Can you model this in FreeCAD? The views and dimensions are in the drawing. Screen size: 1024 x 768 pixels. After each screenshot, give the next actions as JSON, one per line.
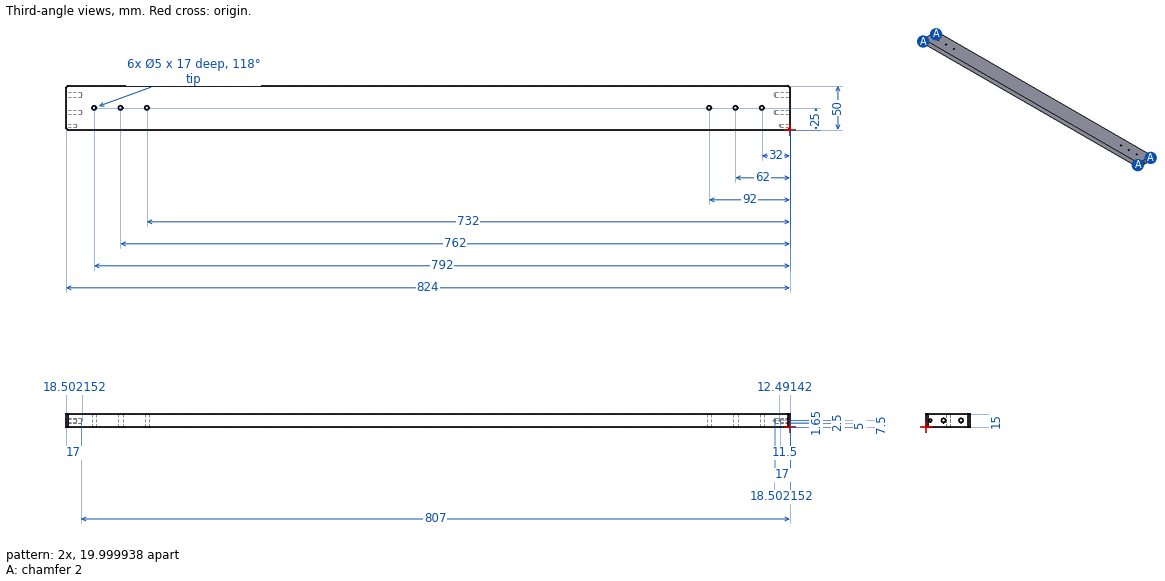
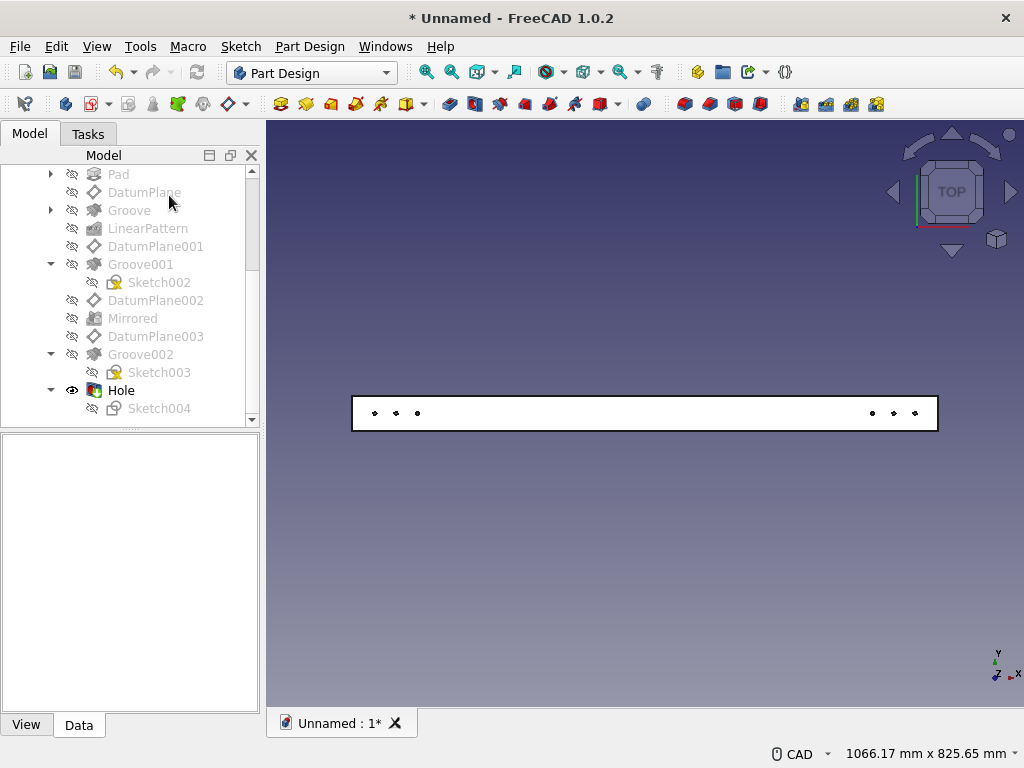
{"action": "key", "text": "1"}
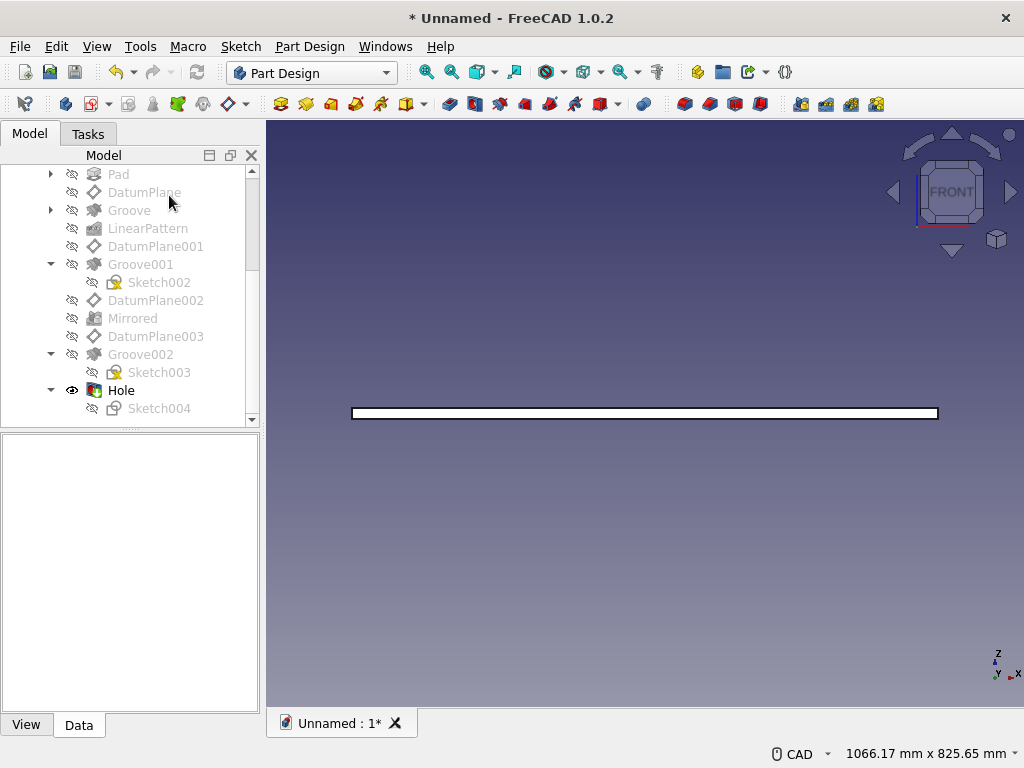
{"action": "key", "text": "3"}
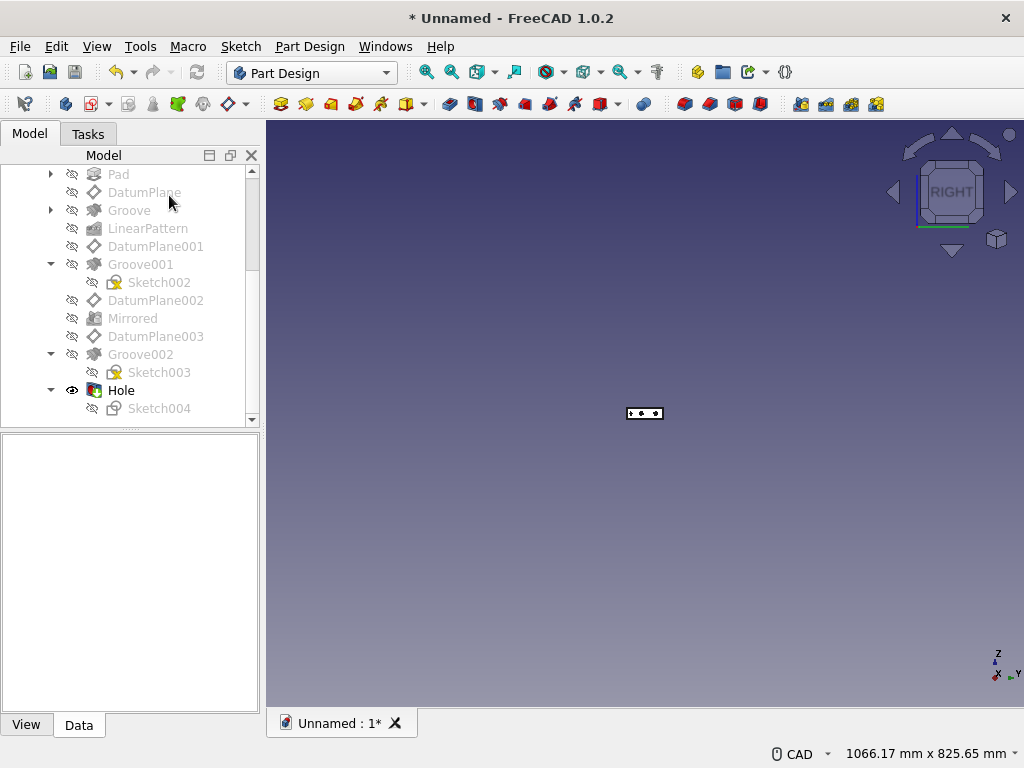
{"action": "left_click", "coordinate": [427, 72]}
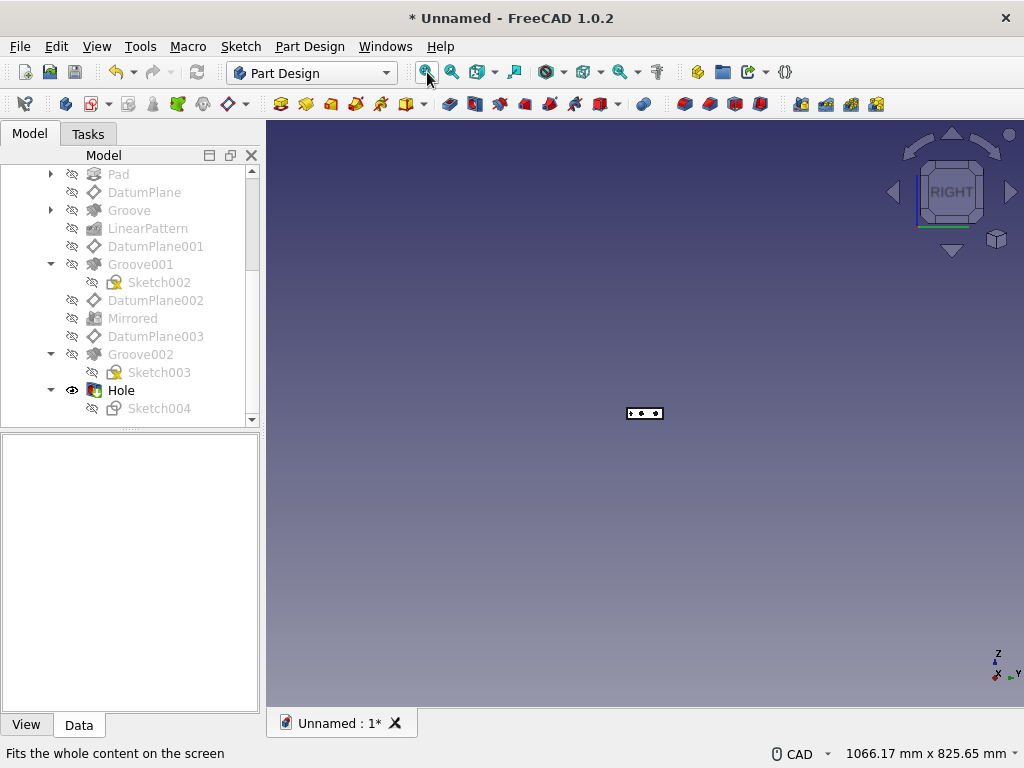
{"action": "scroll", "coordinate": [663, 412], "scroll_direction": "up", "scroll_amount": 7}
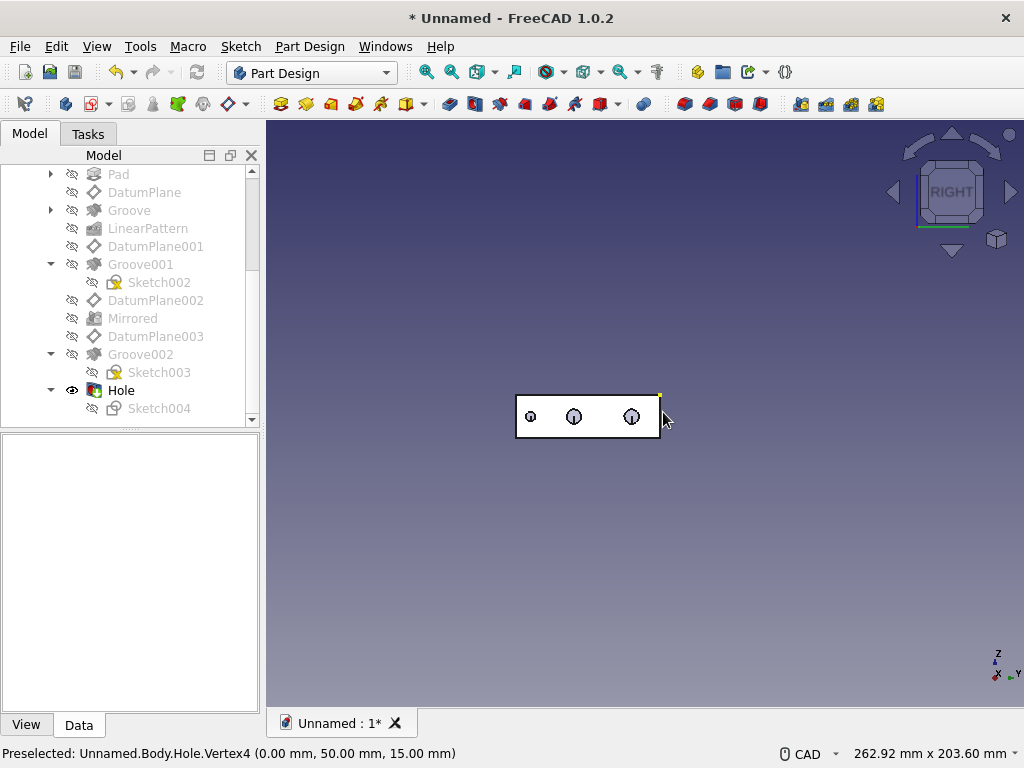
{"action": "left_click", "coordinate": [660, 416]}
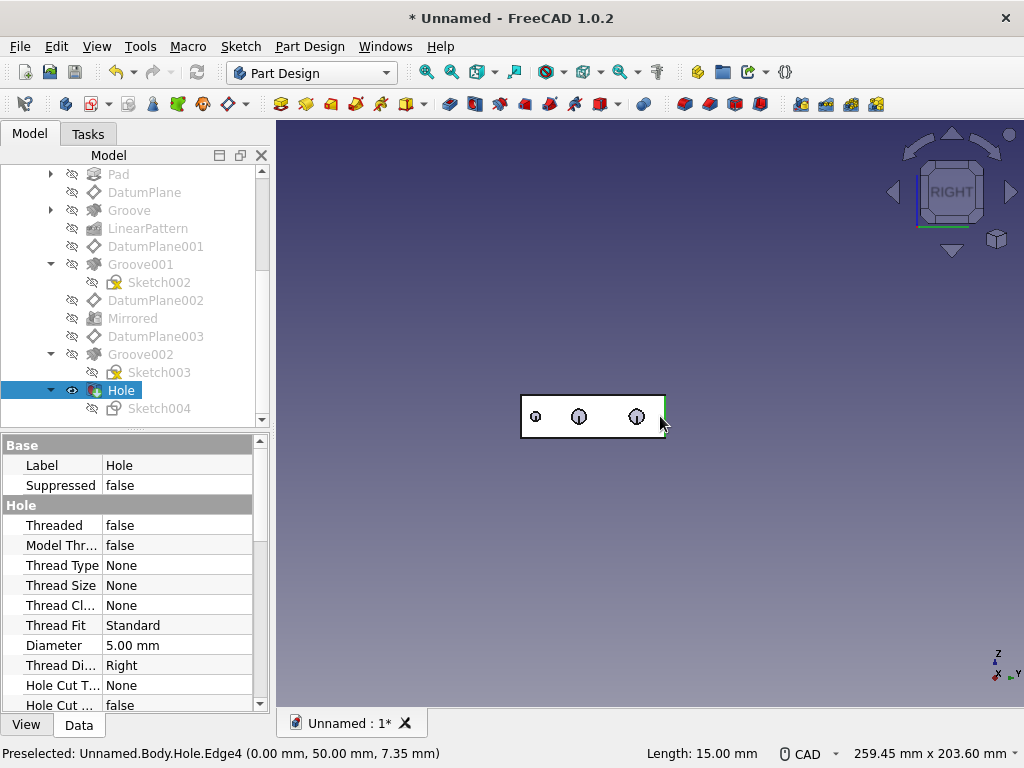
{"action": "left_click", "coordinate": [521, 416], "text": "ctrl"}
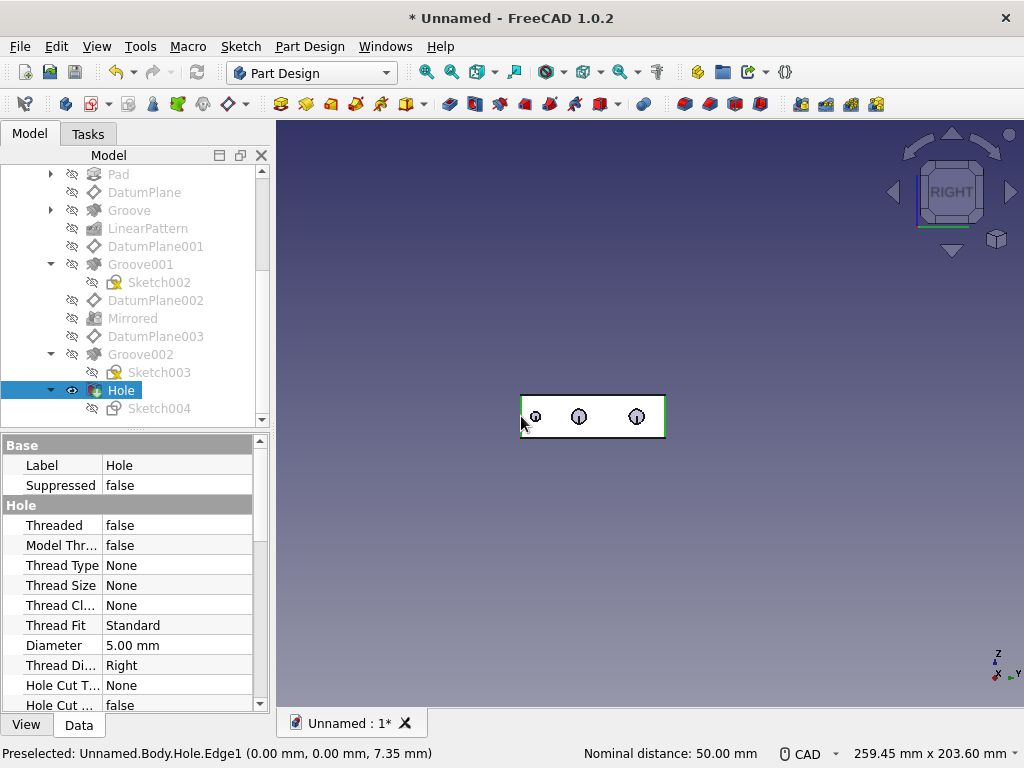
{"action": "left_click", "coordinate": [427, 72]}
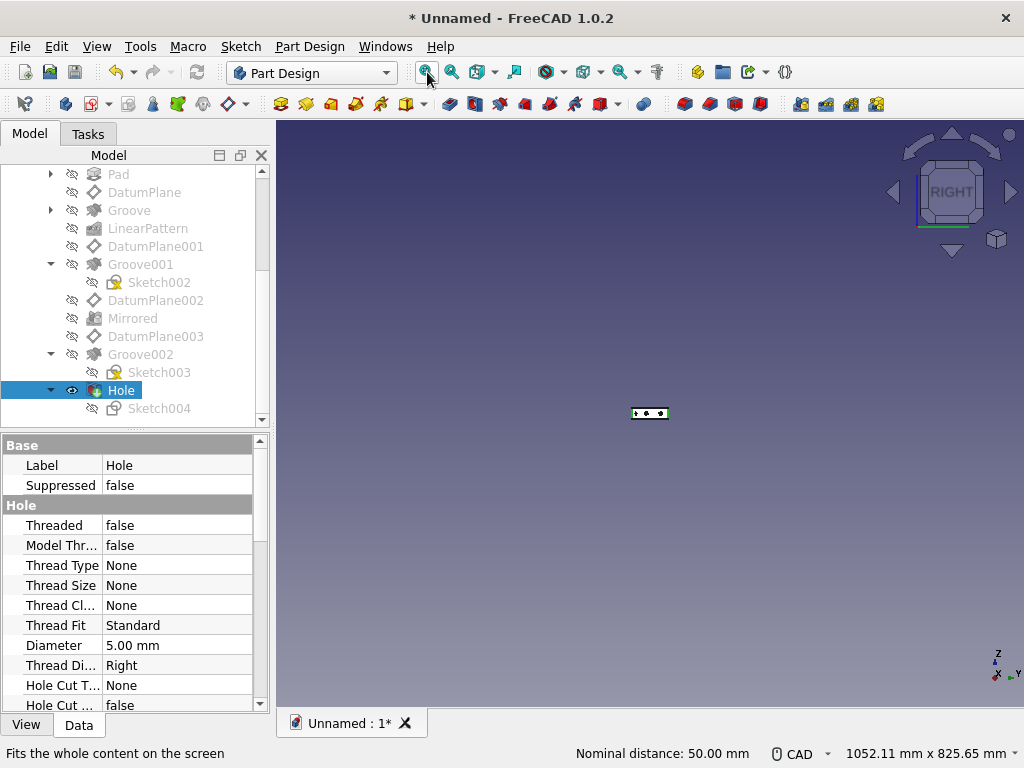
{"action": "key", "text": "5"}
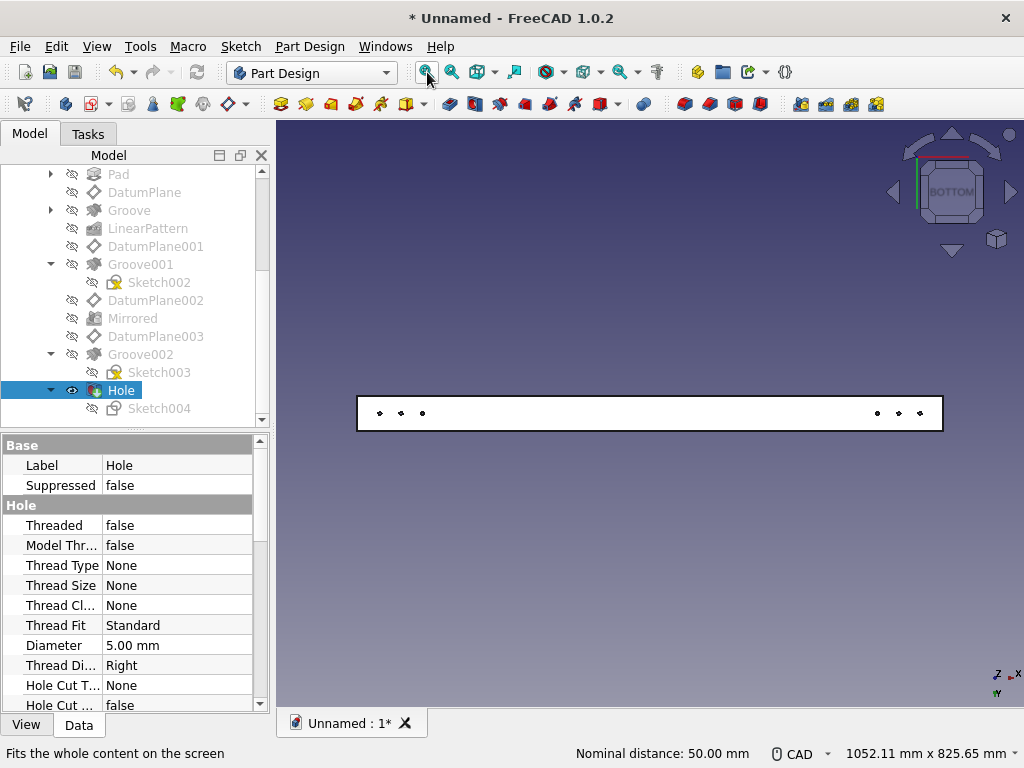
{"action": "scroll", "coordinate": [357, 395], "scroll_direction": "up", "scroll_amount": 7}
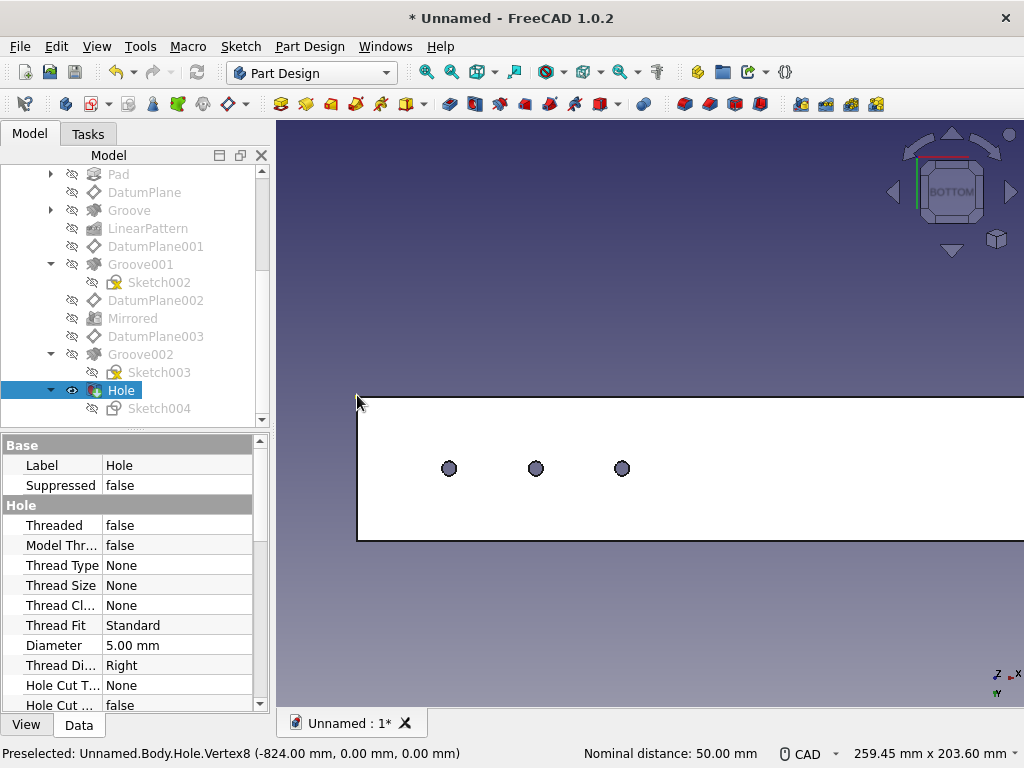
{"action": "left_click", "coordinate": [427, 72]}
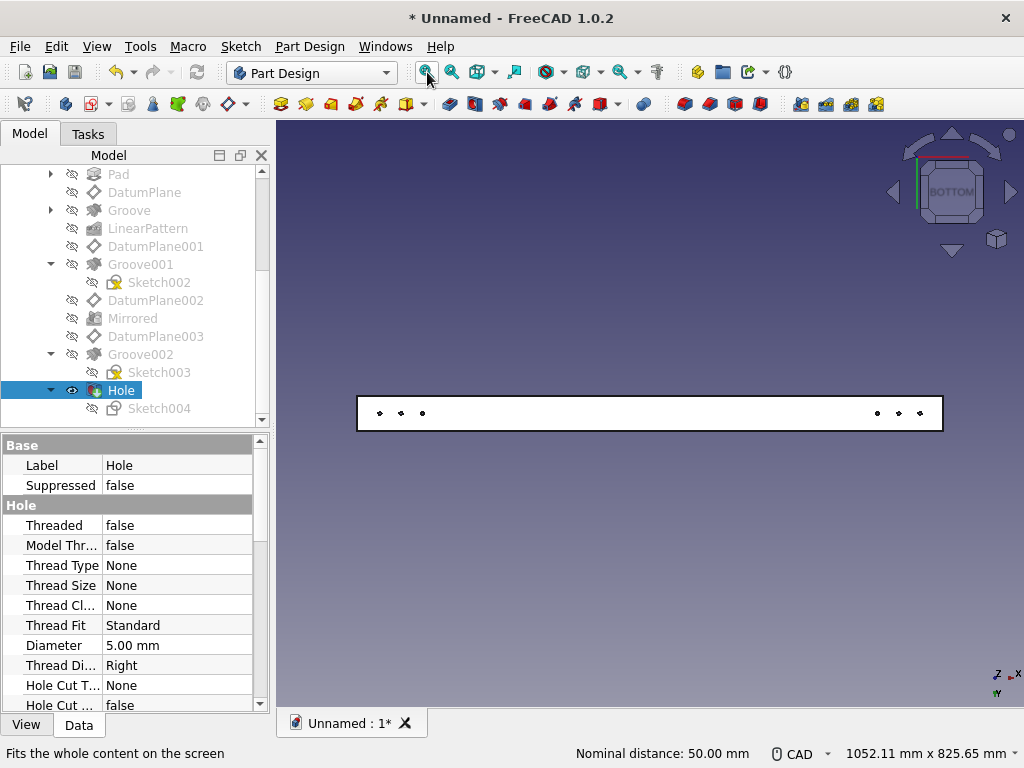
{"action": "key", "text": "4"}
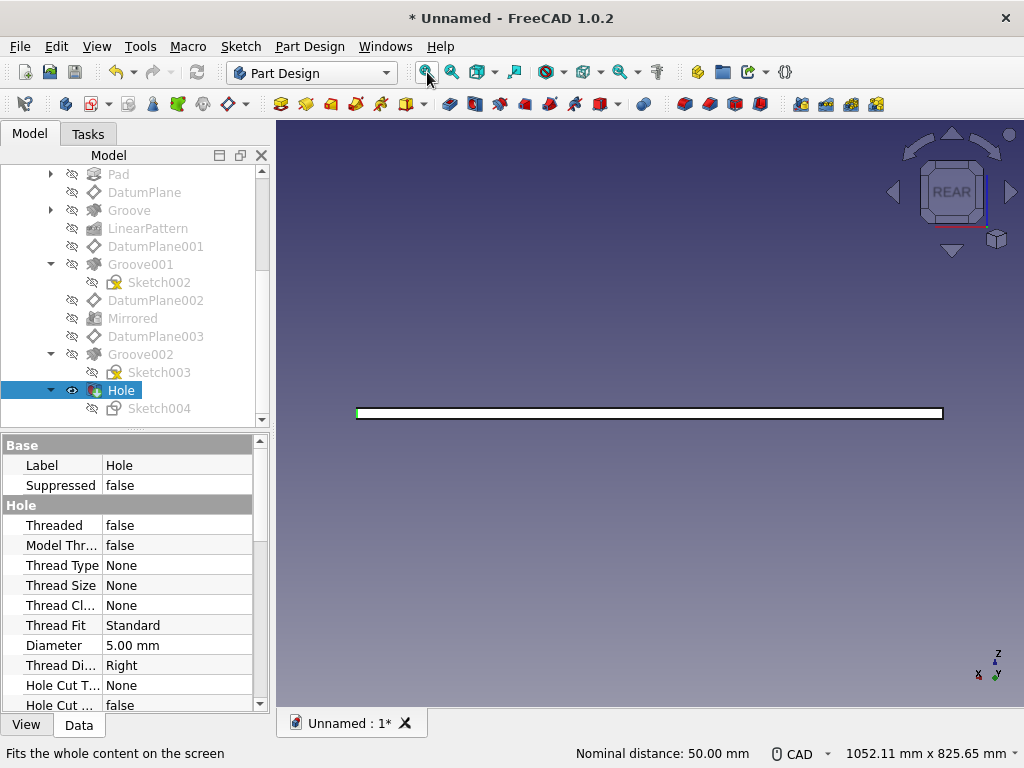
{"action": "key", "text": "6"}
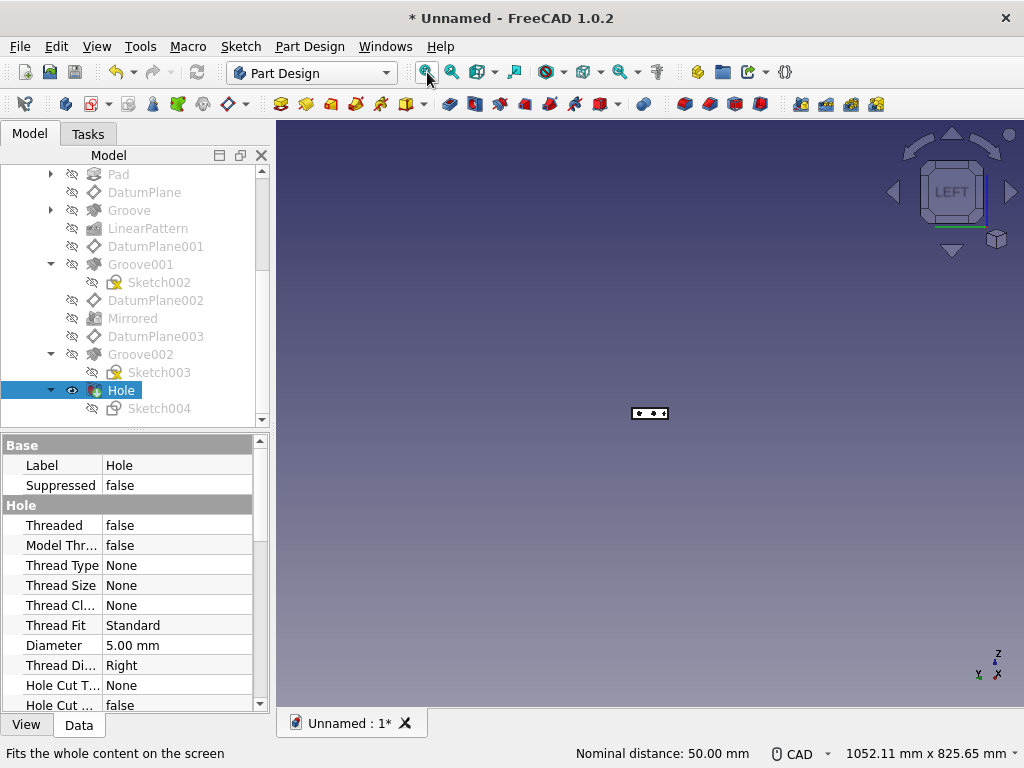
{"action": "left_click", "coordinate": [427, 72]}